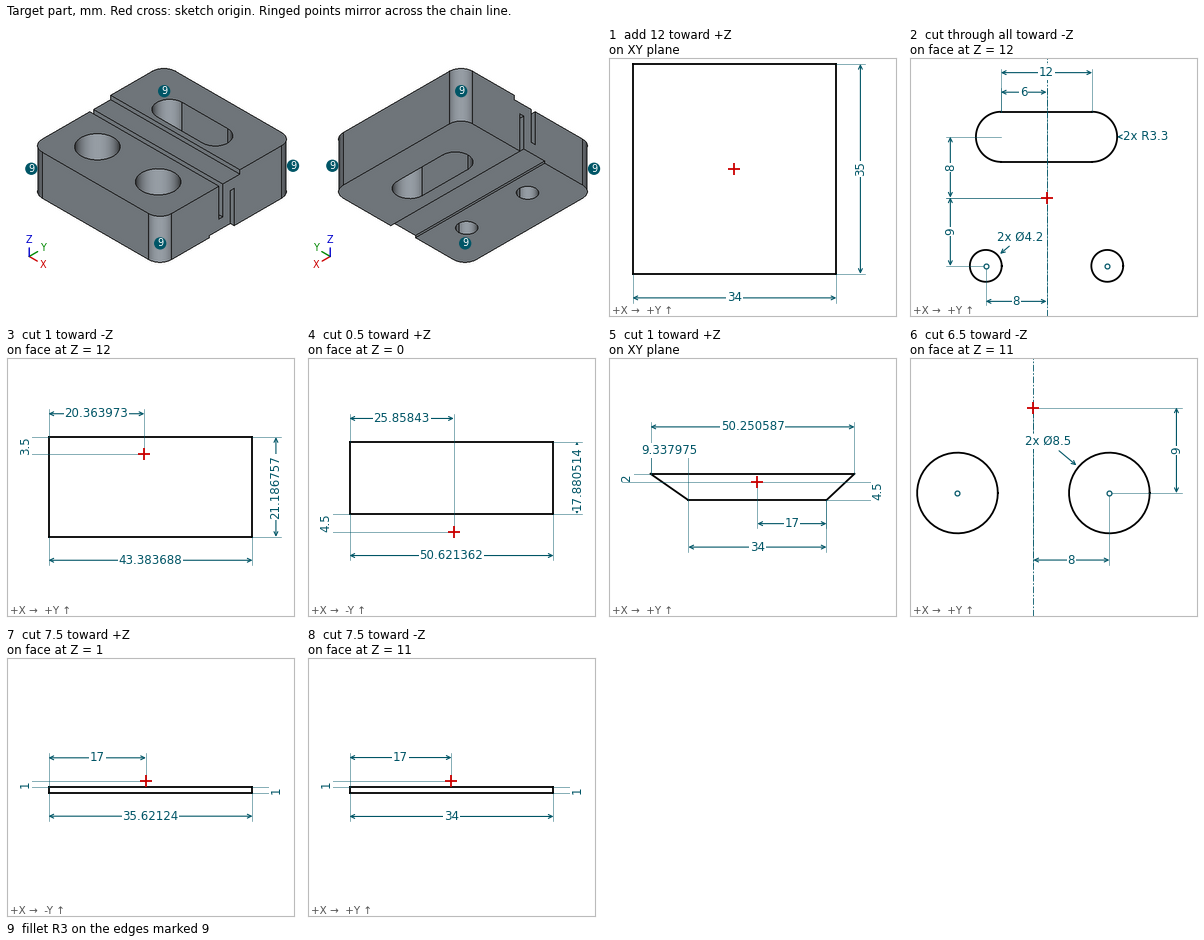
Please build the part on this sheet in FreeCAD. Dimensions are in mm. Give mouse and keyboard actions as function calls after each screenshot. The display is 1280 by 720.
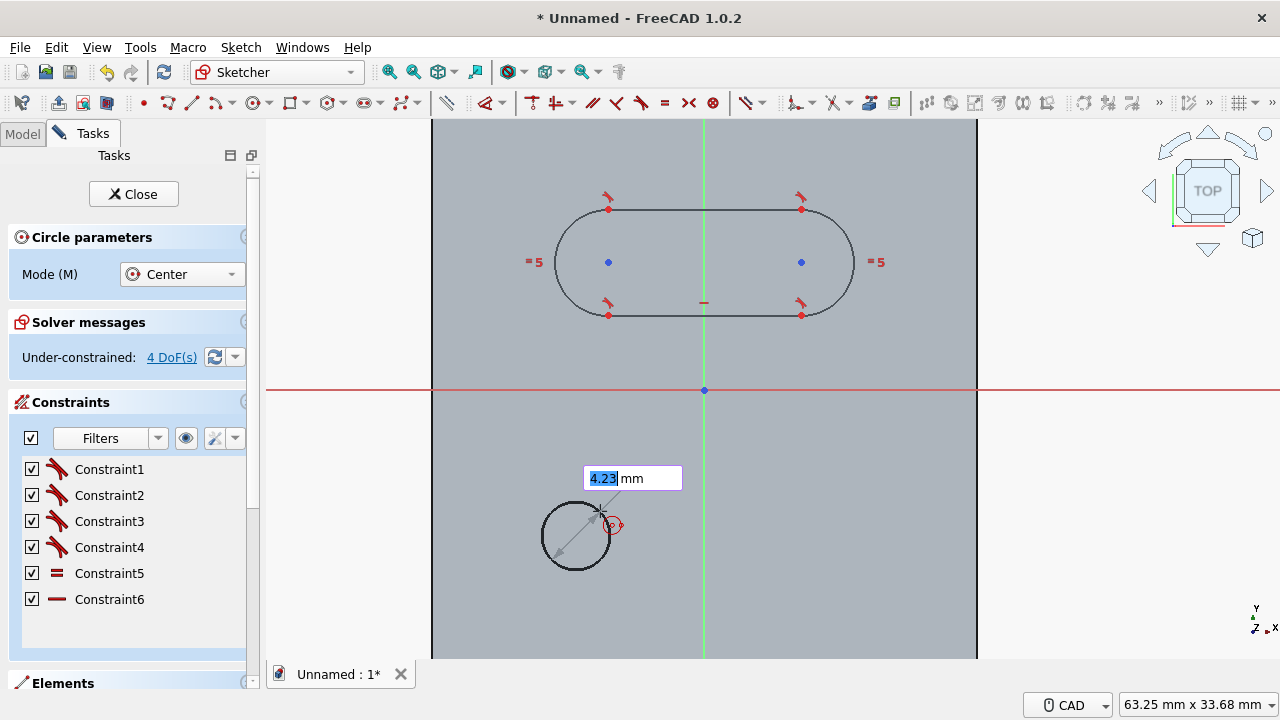
text(4.2)
key(Return)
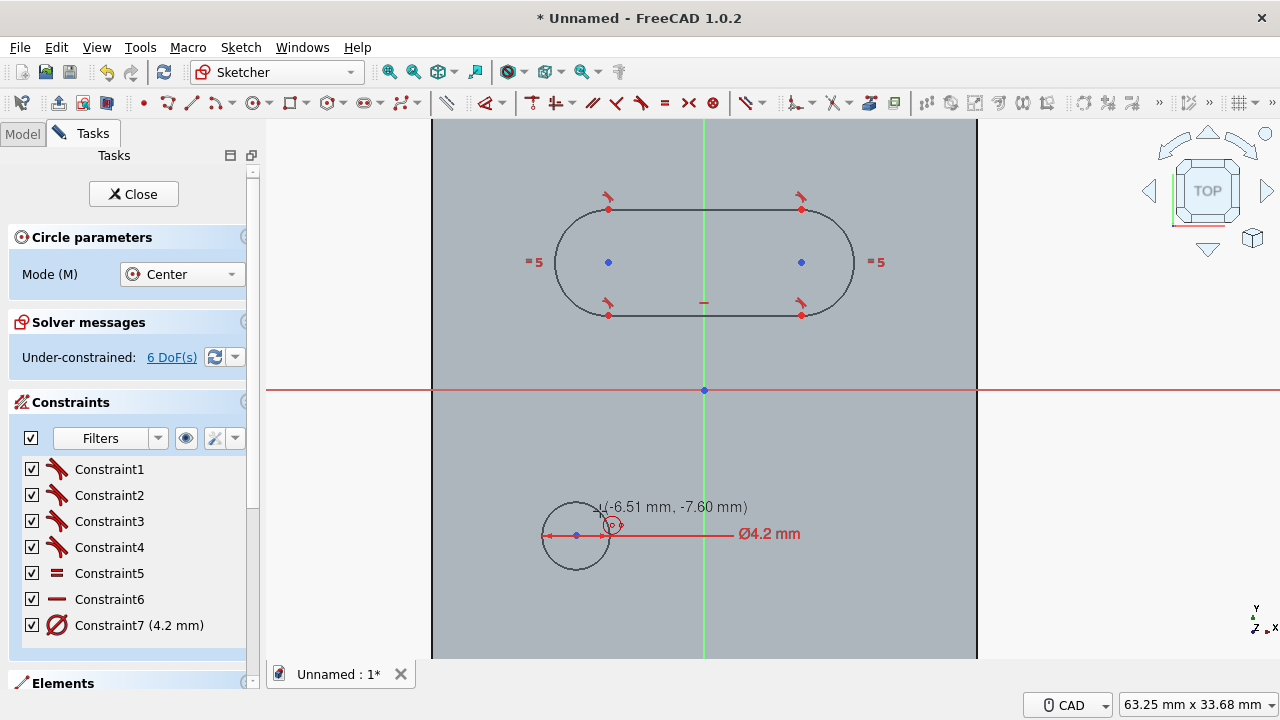
click(833, 535)
move(856, 511)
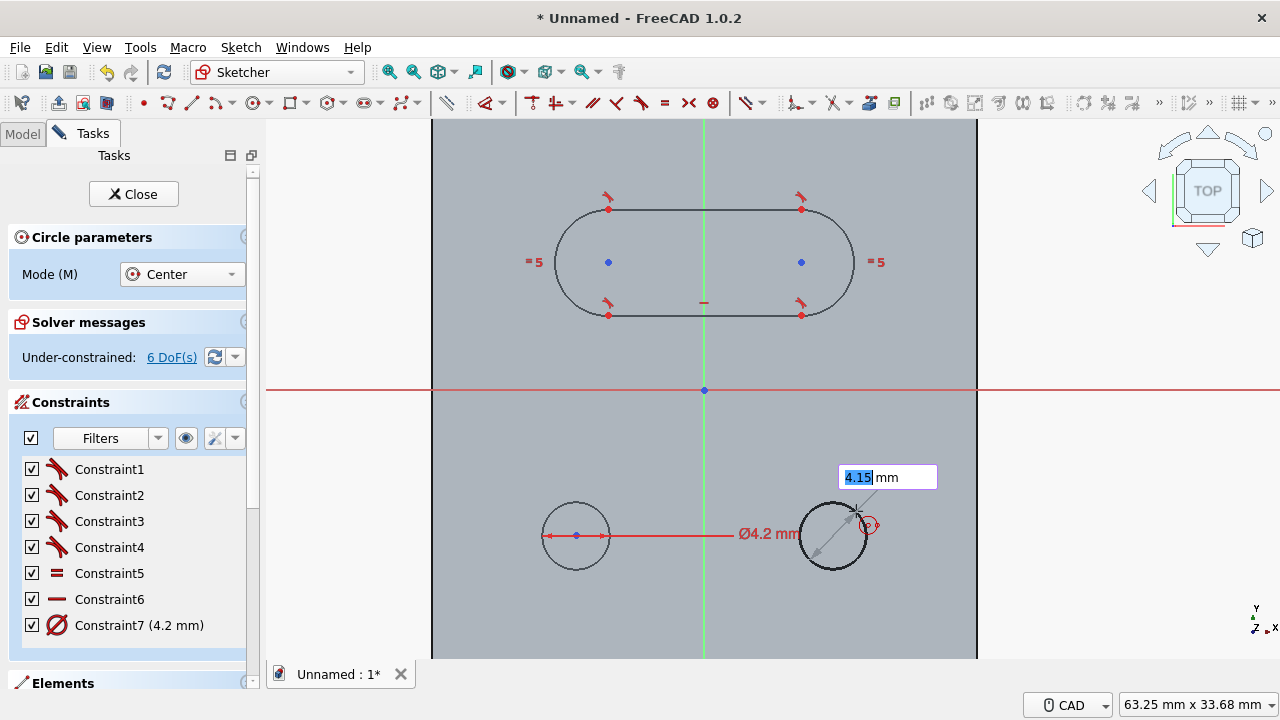
text(4.2)
key(Return)
key(Escape)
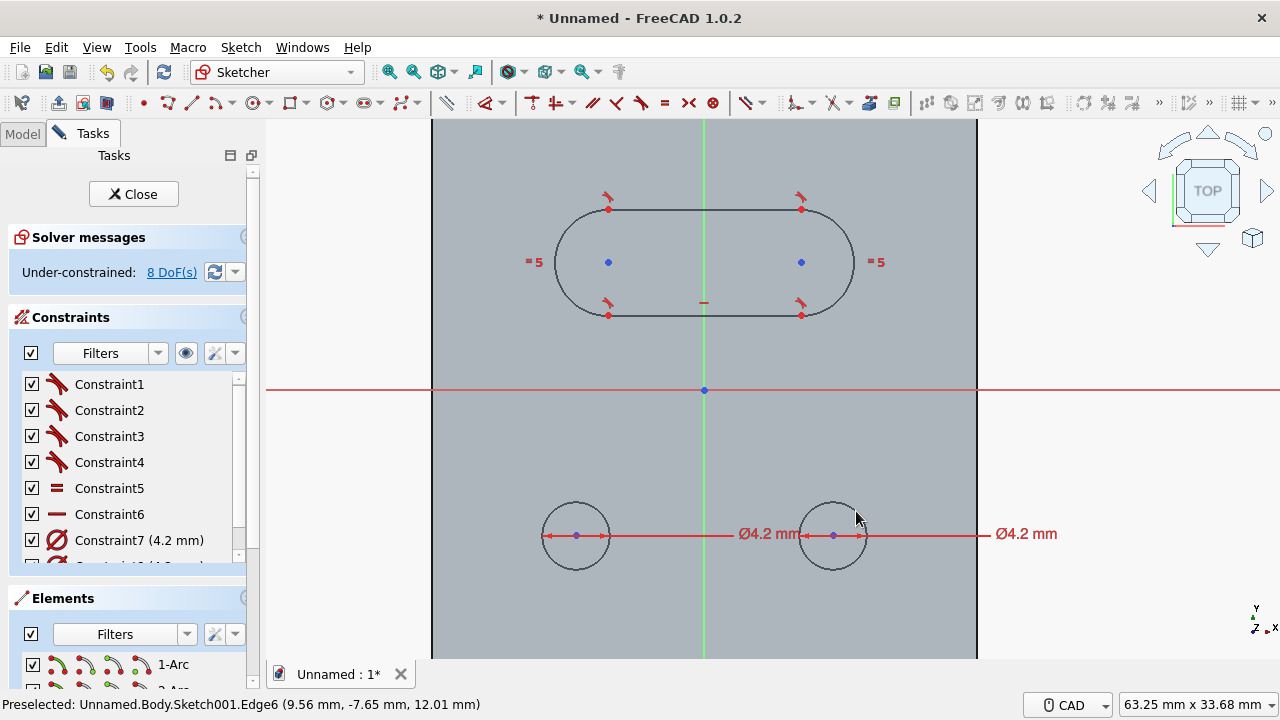
click(576, 536)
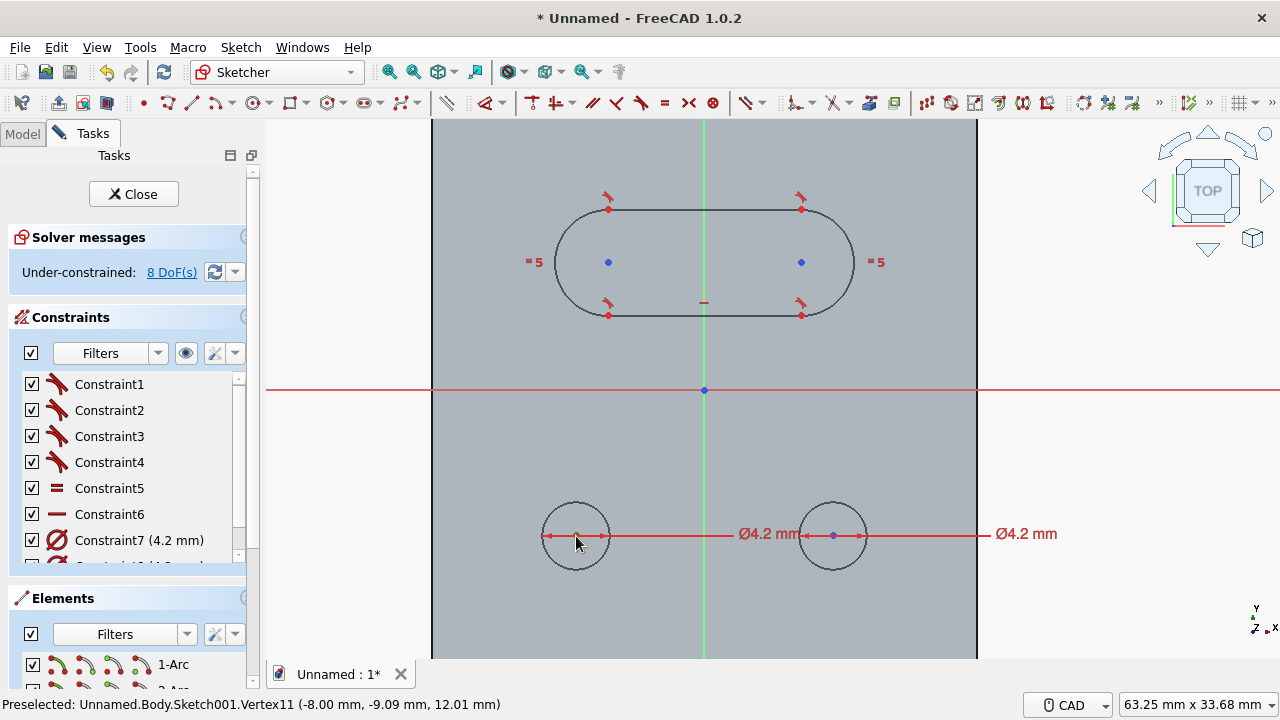
click(833, 536)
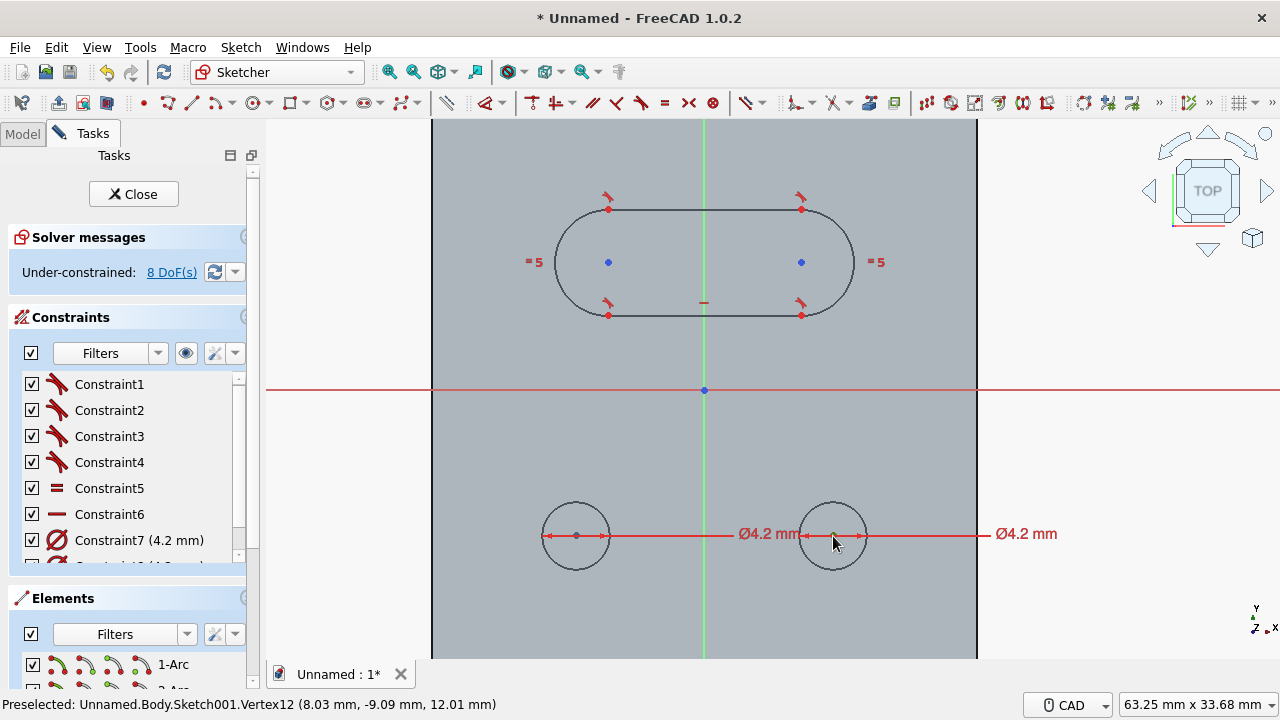
click(704, 596)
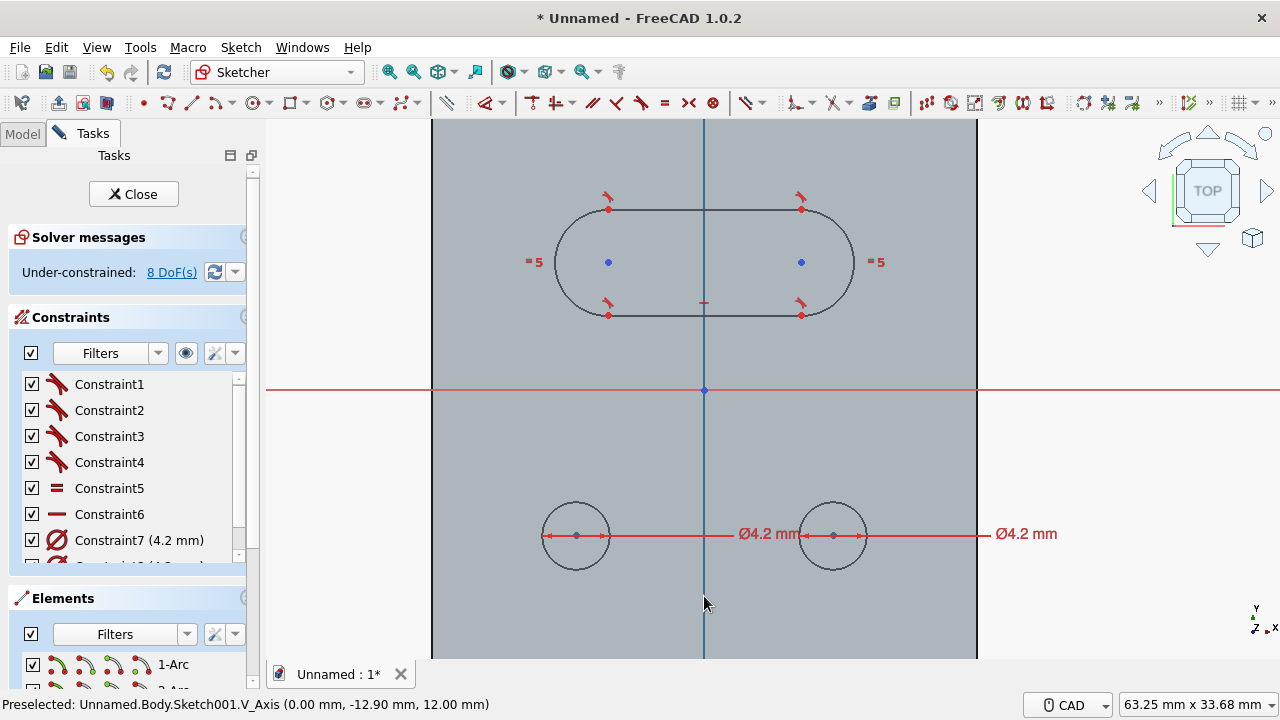
key(s)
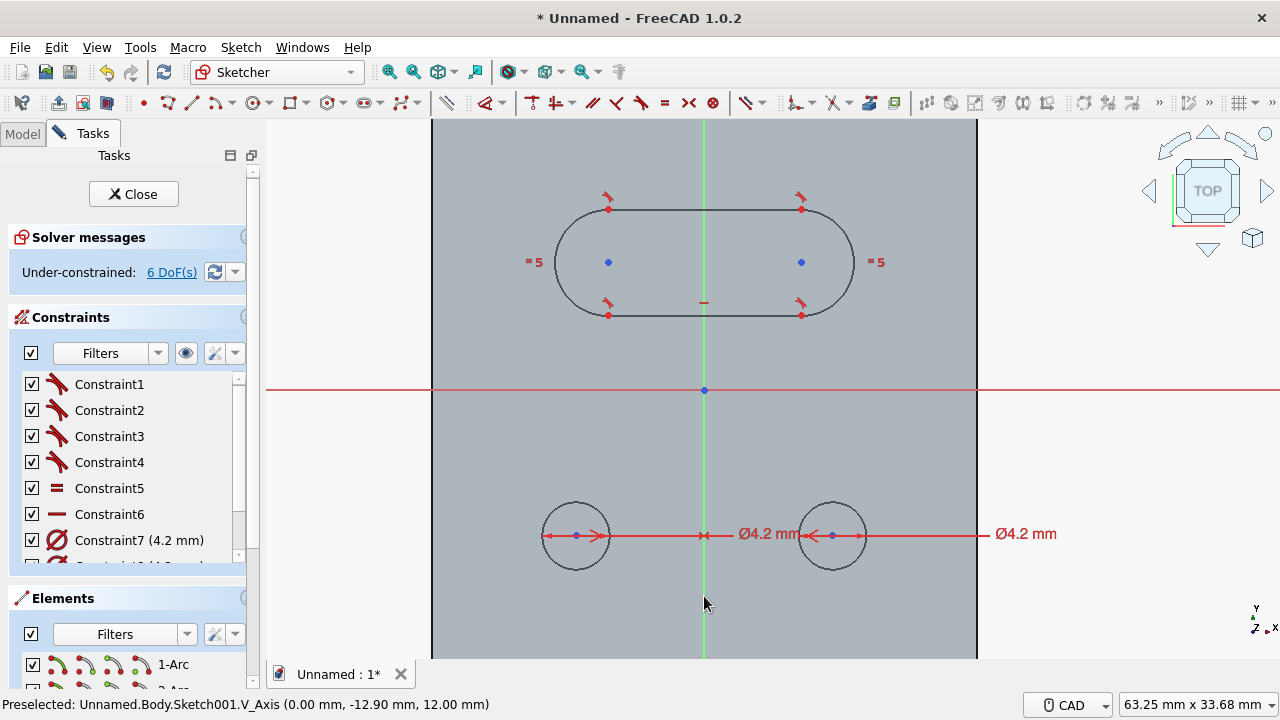
key(d)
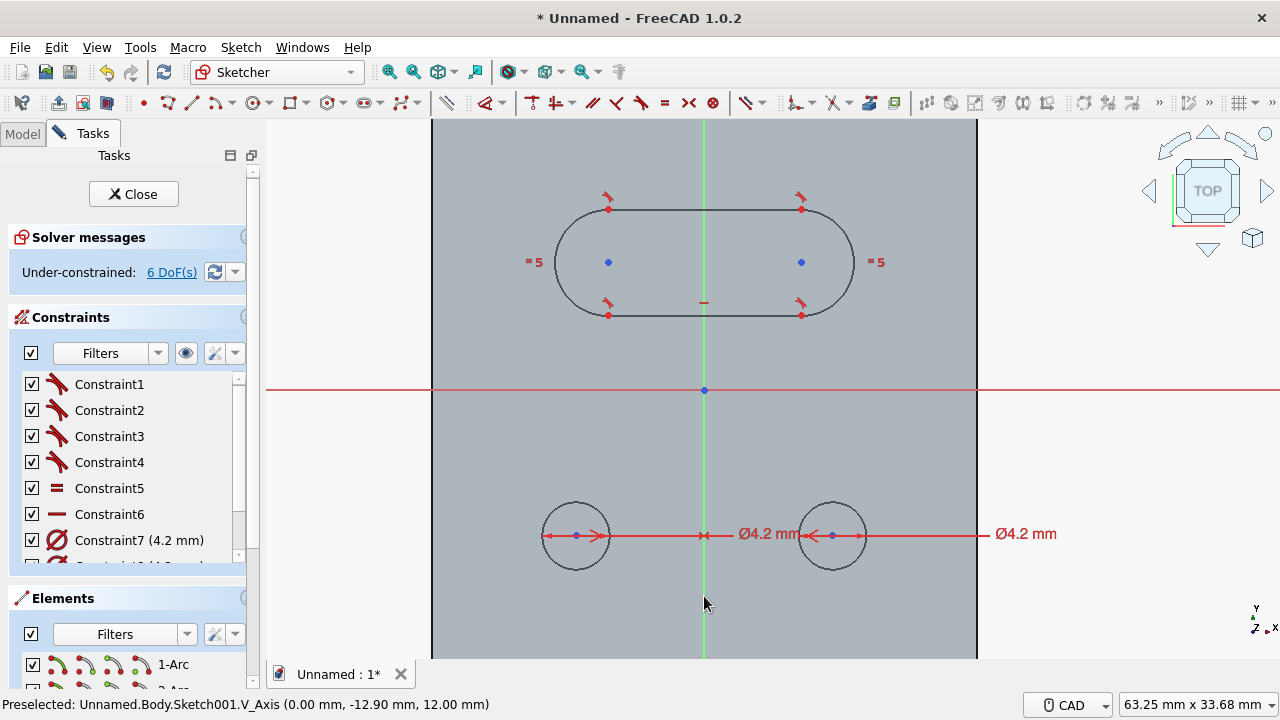
click(565, 232)
click(539, 213)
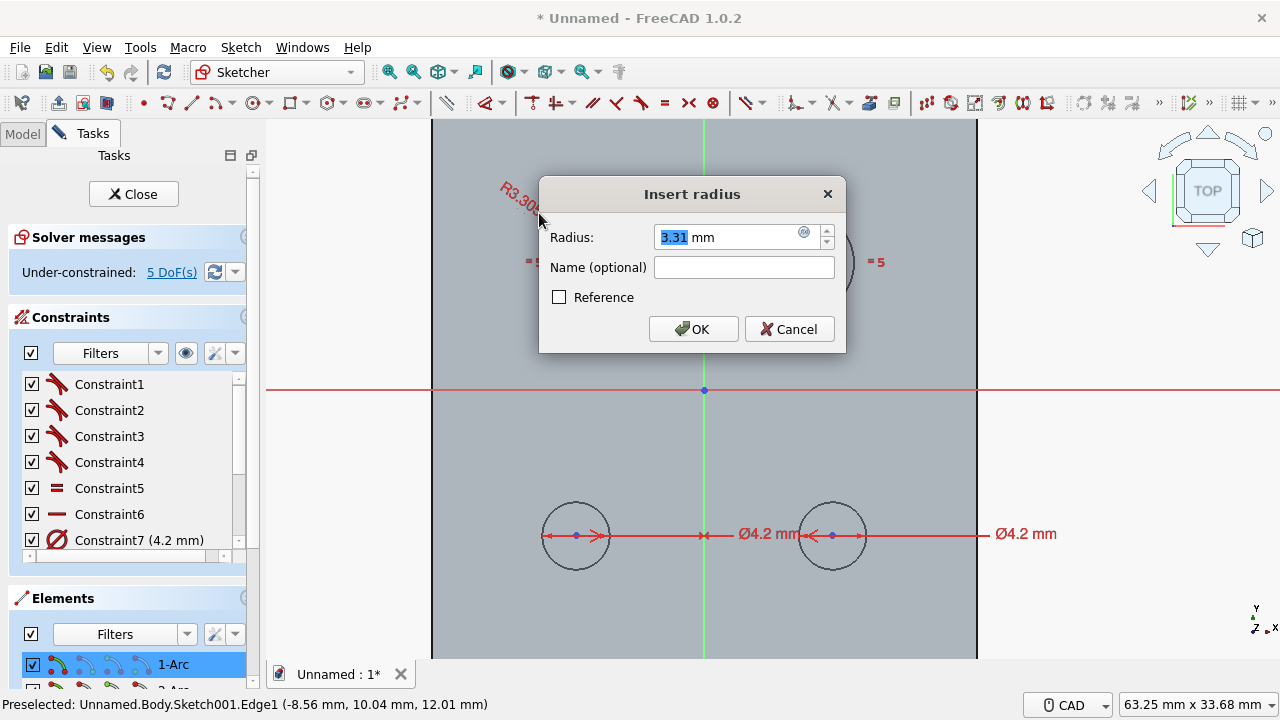
text(3.3)
key(Return)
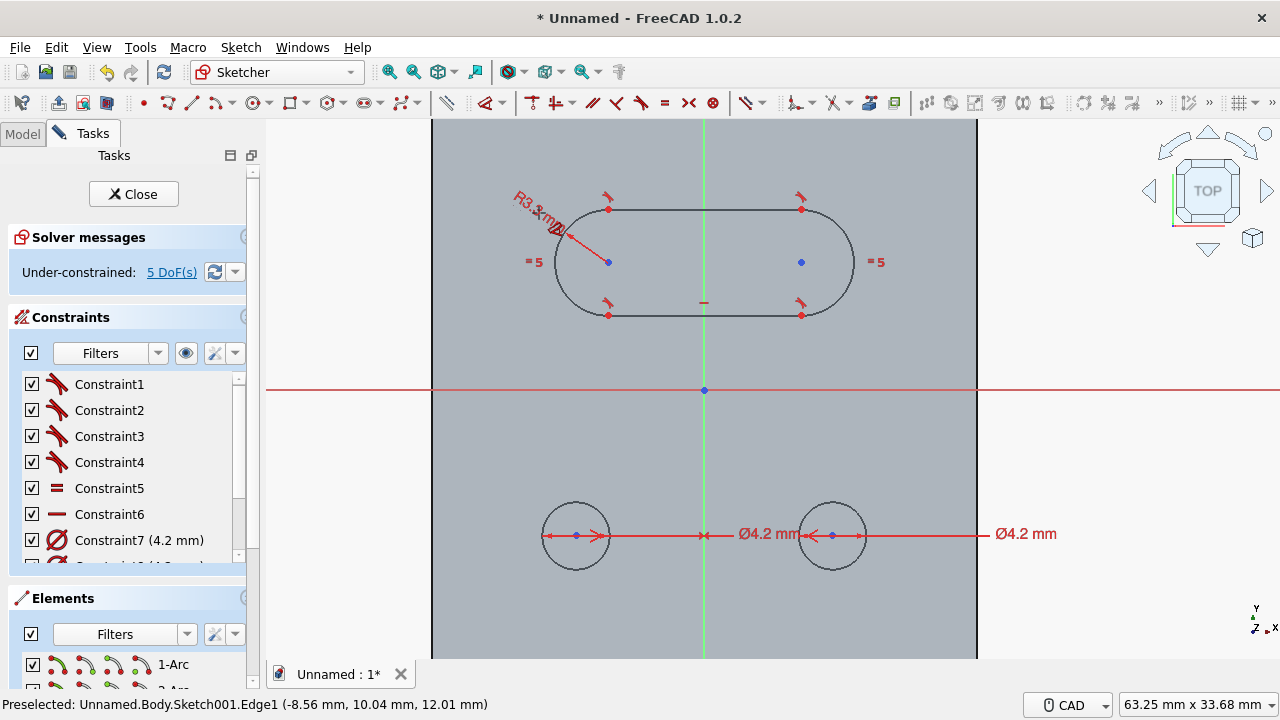
click(576, 536)
click(640, 570)